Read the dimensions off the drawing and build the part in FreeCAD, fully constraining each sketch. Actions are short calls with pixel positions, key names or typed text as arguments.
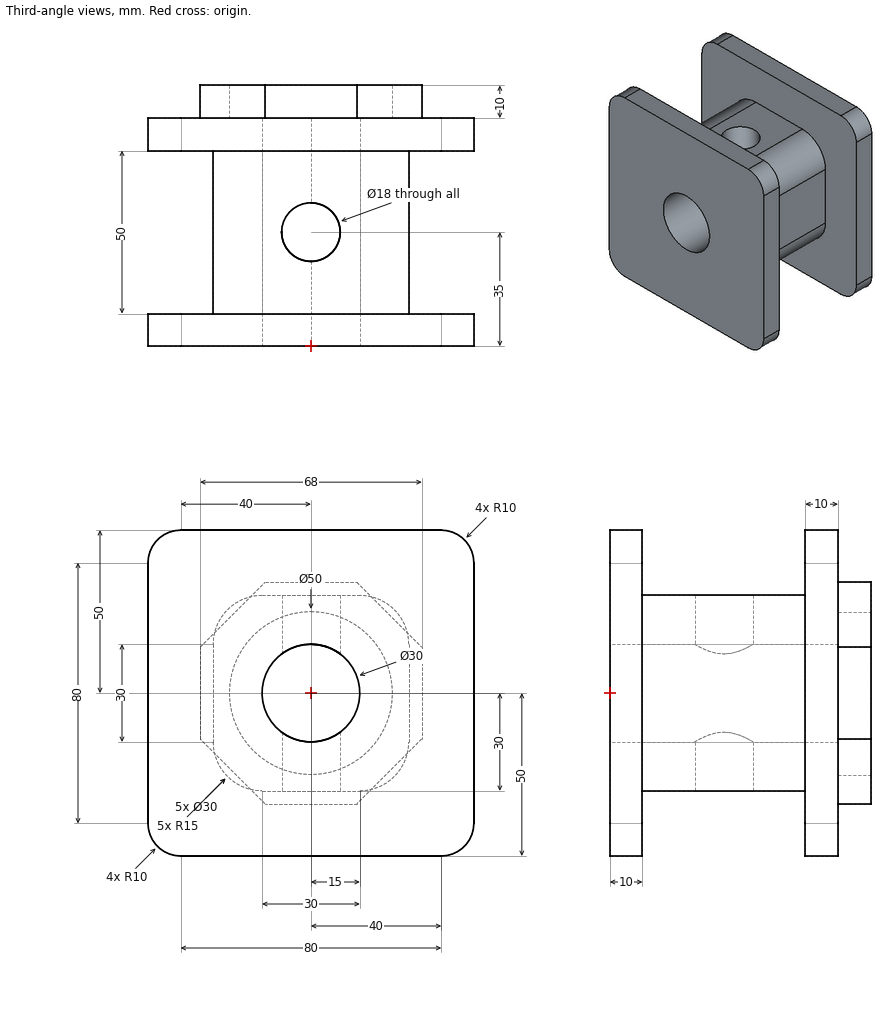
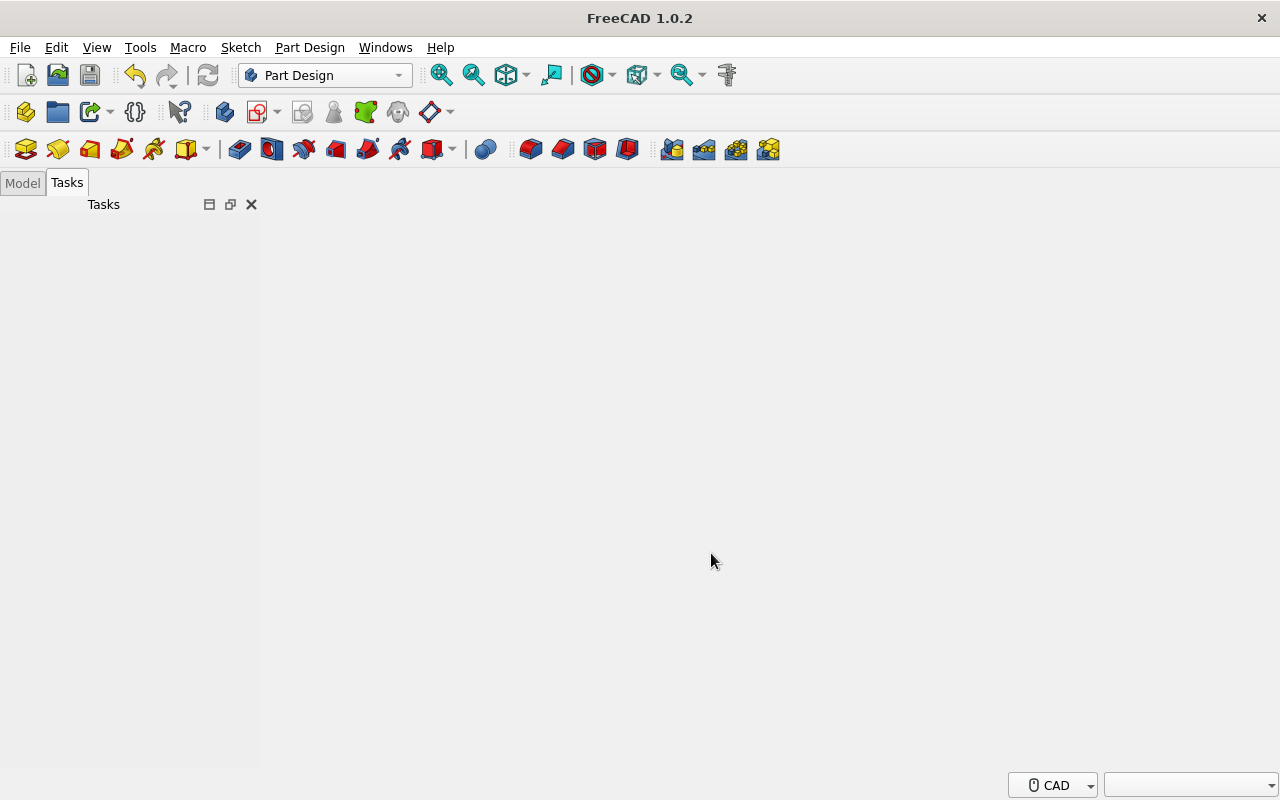
click(26, 76)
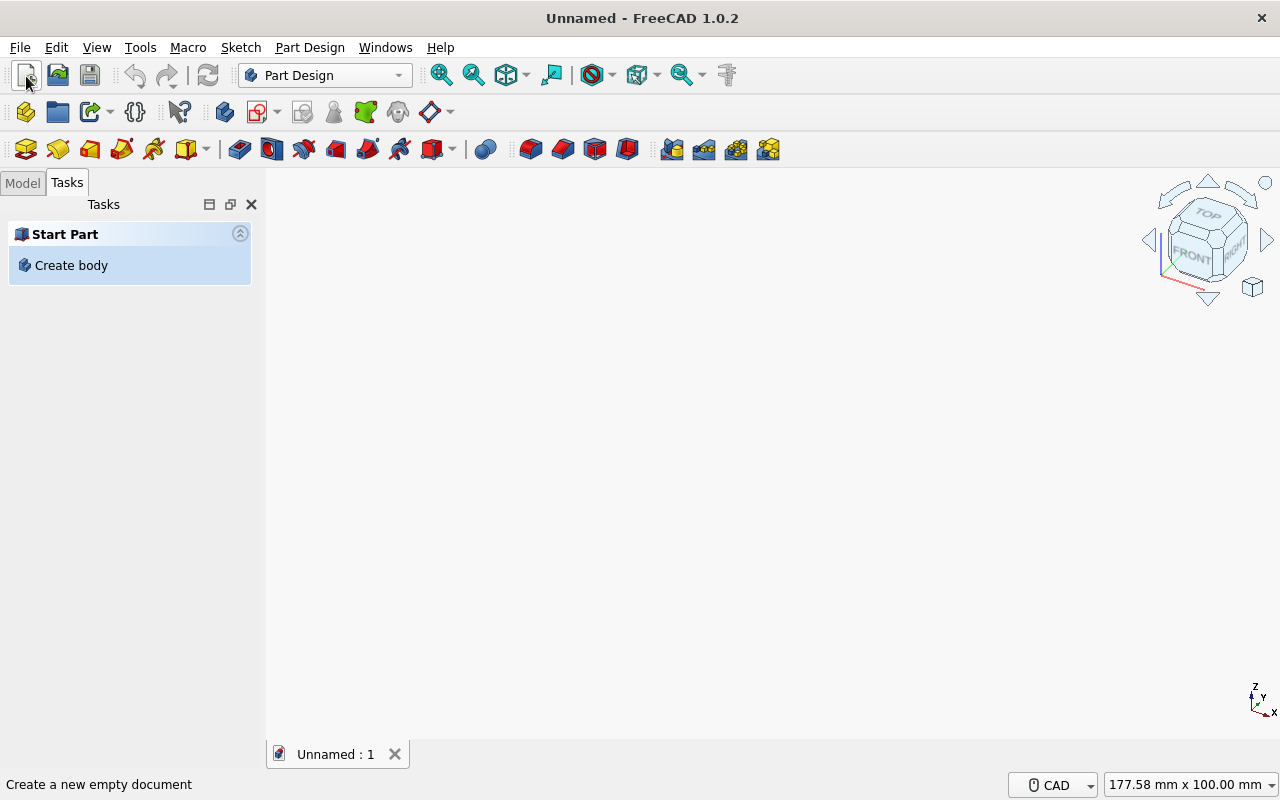
click(258, 112)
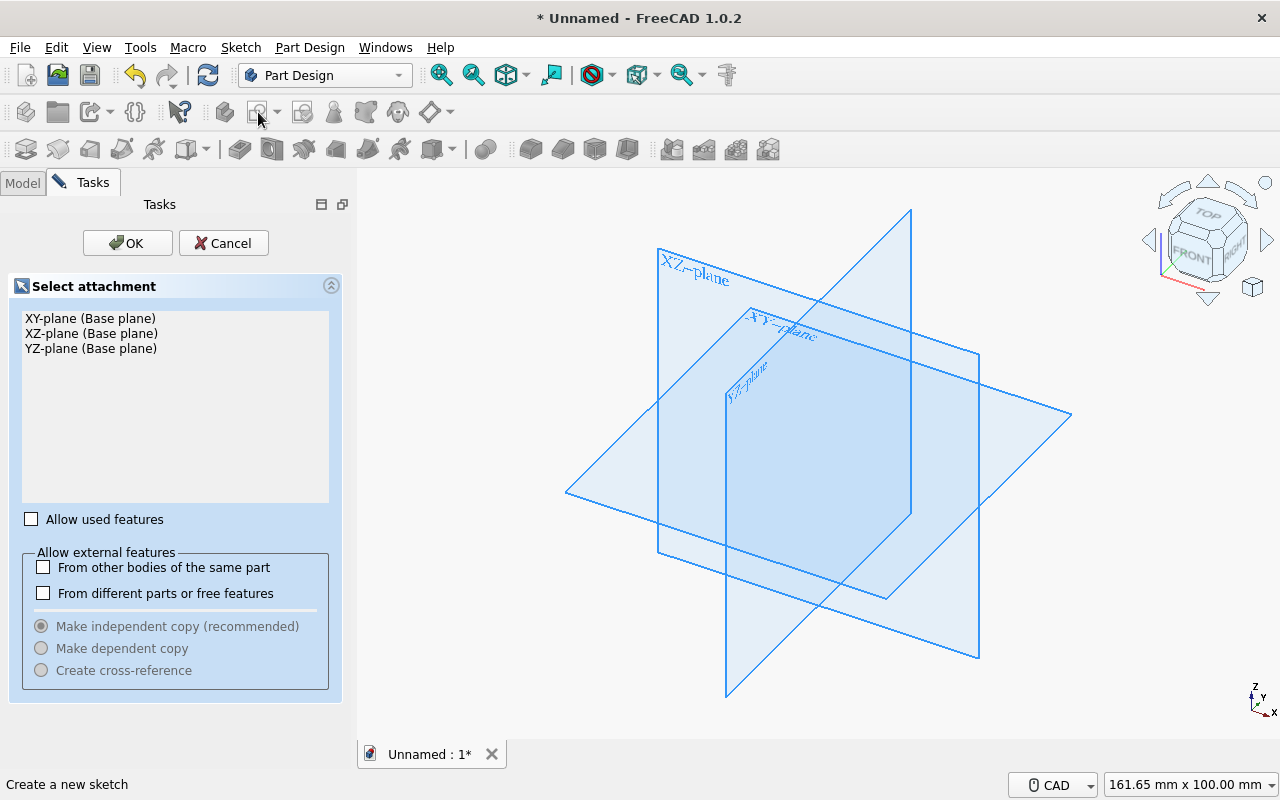
click(82, 334)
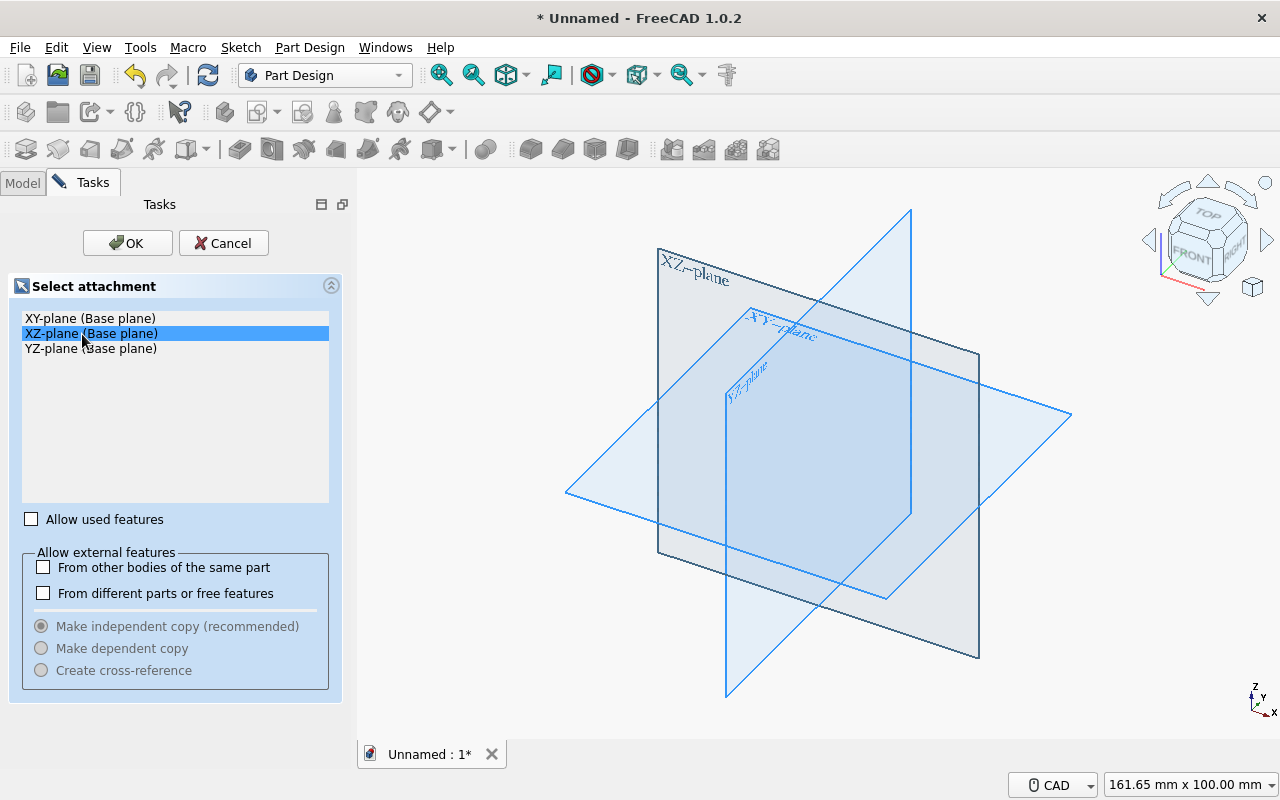
click(128, 243)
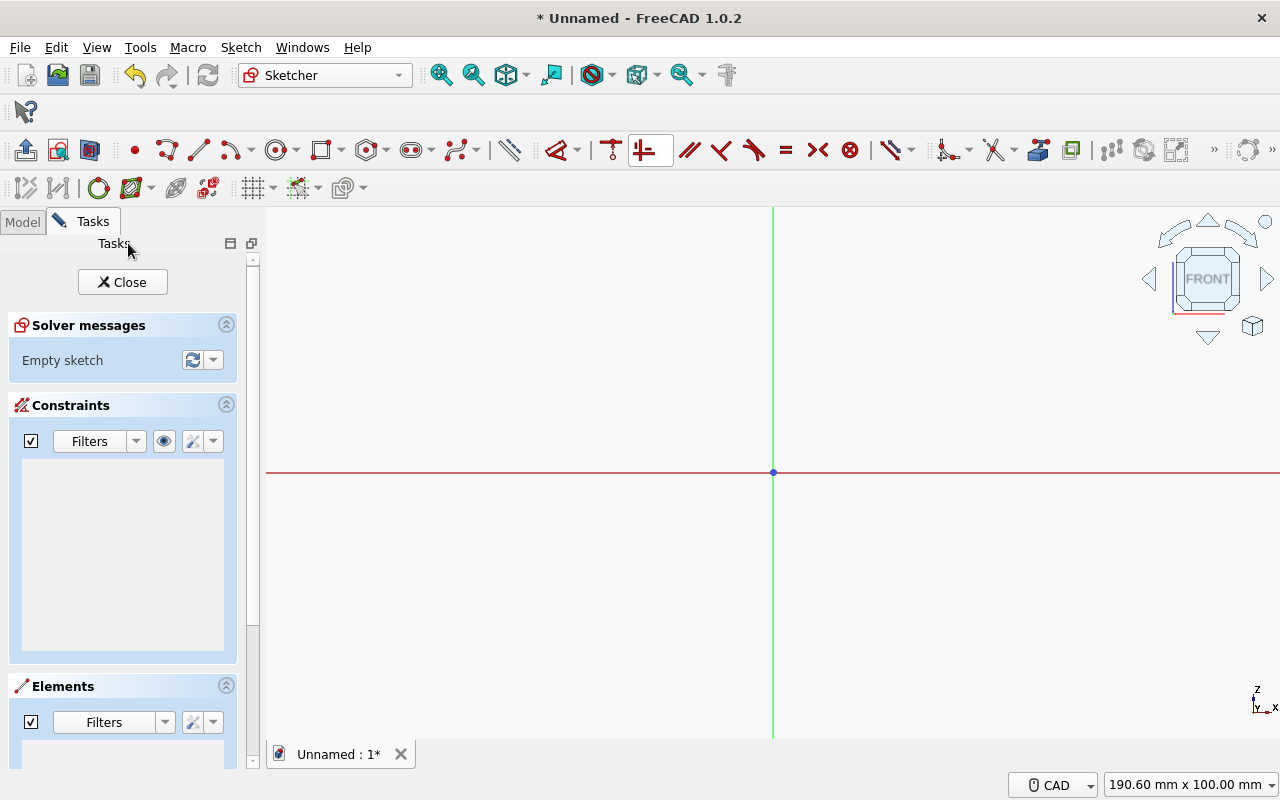
scroll(565, 473, down, 2)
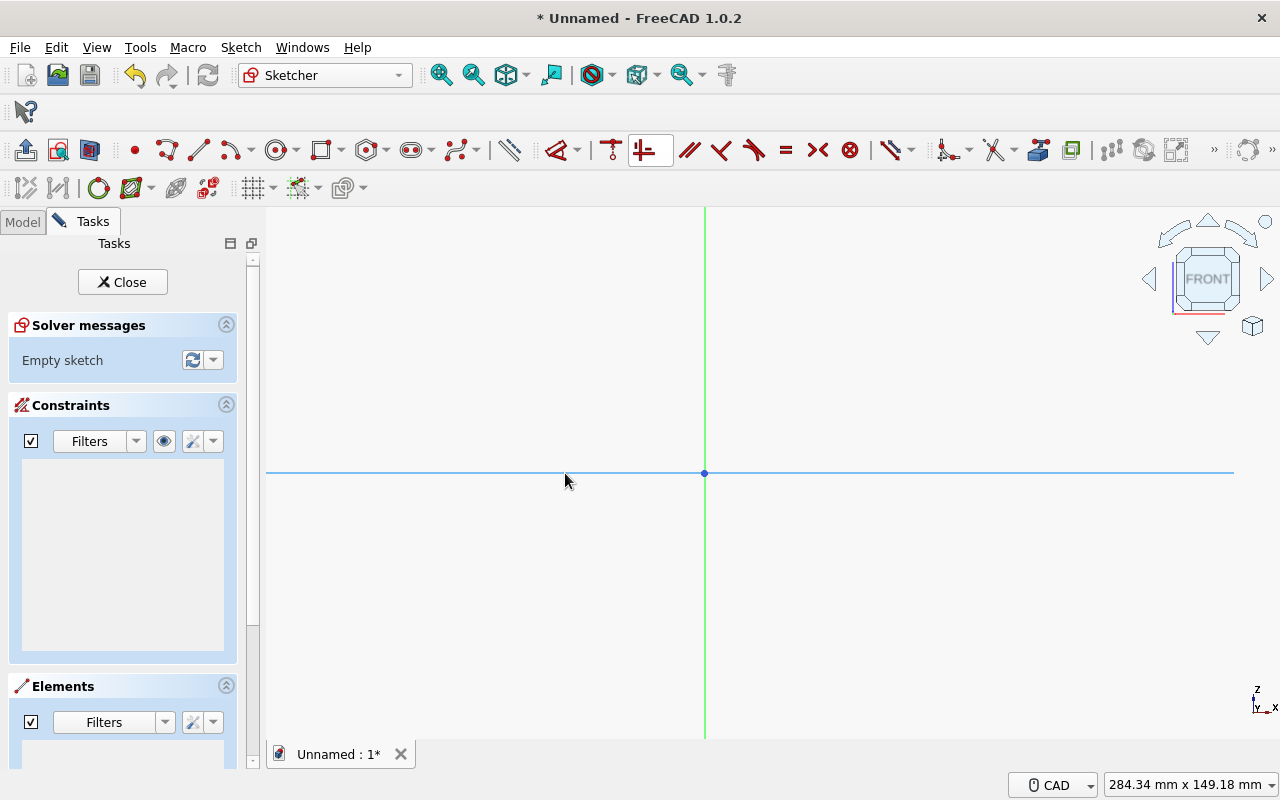
click(200, 150)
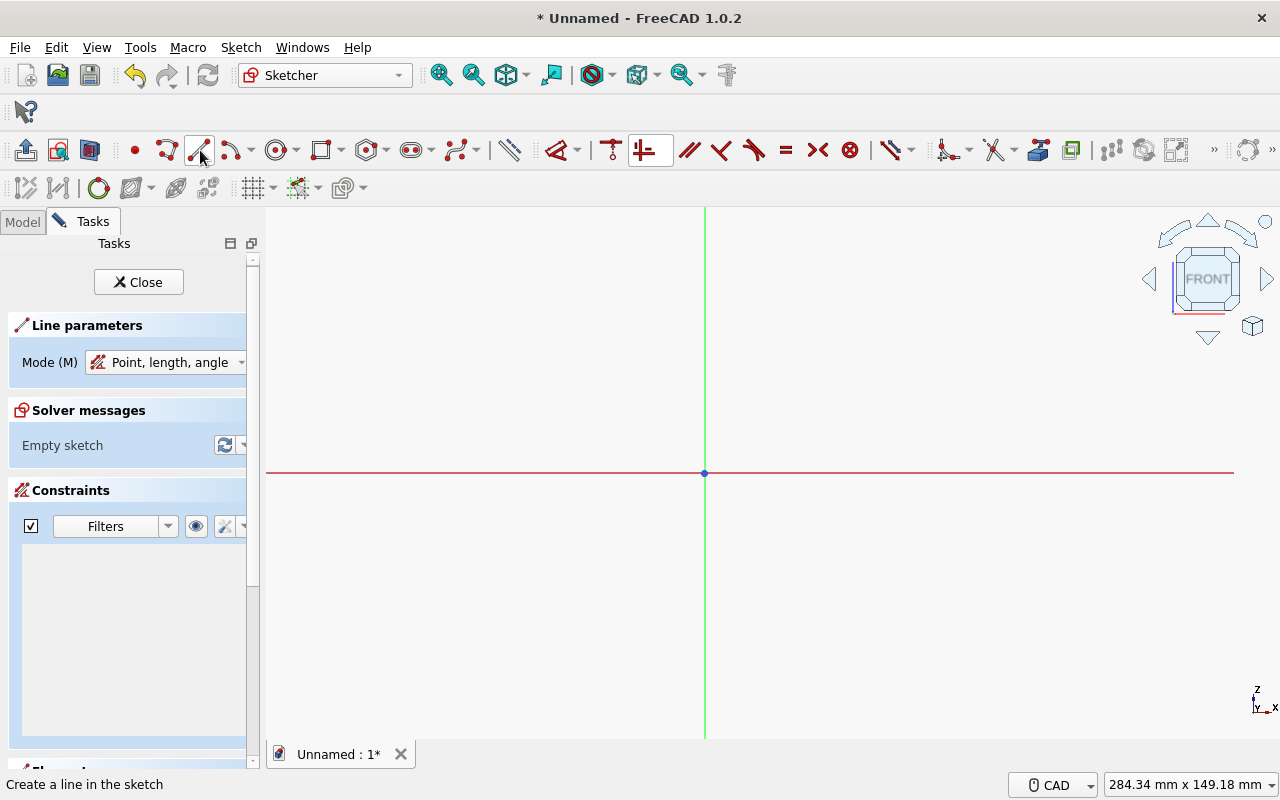
click(847, 651)
click(562, 651)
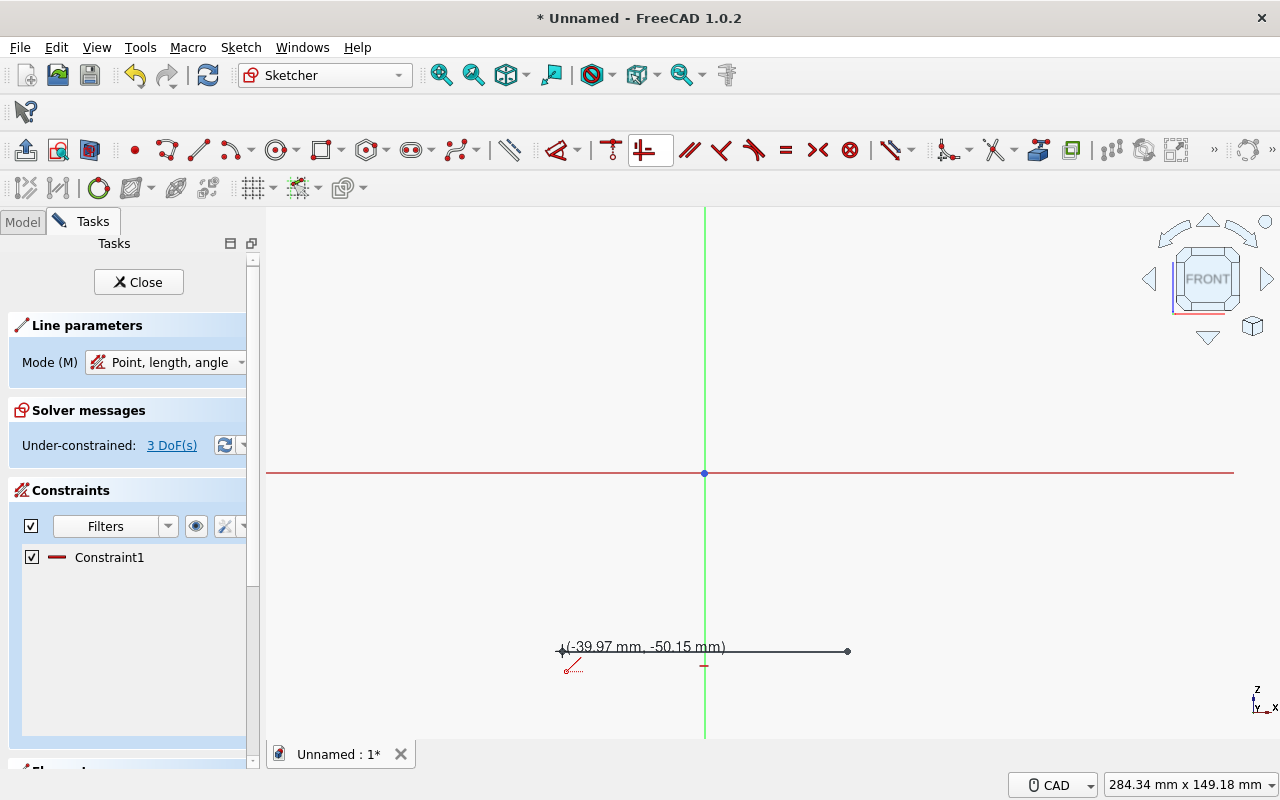
click(526, 616)
click(526, 331)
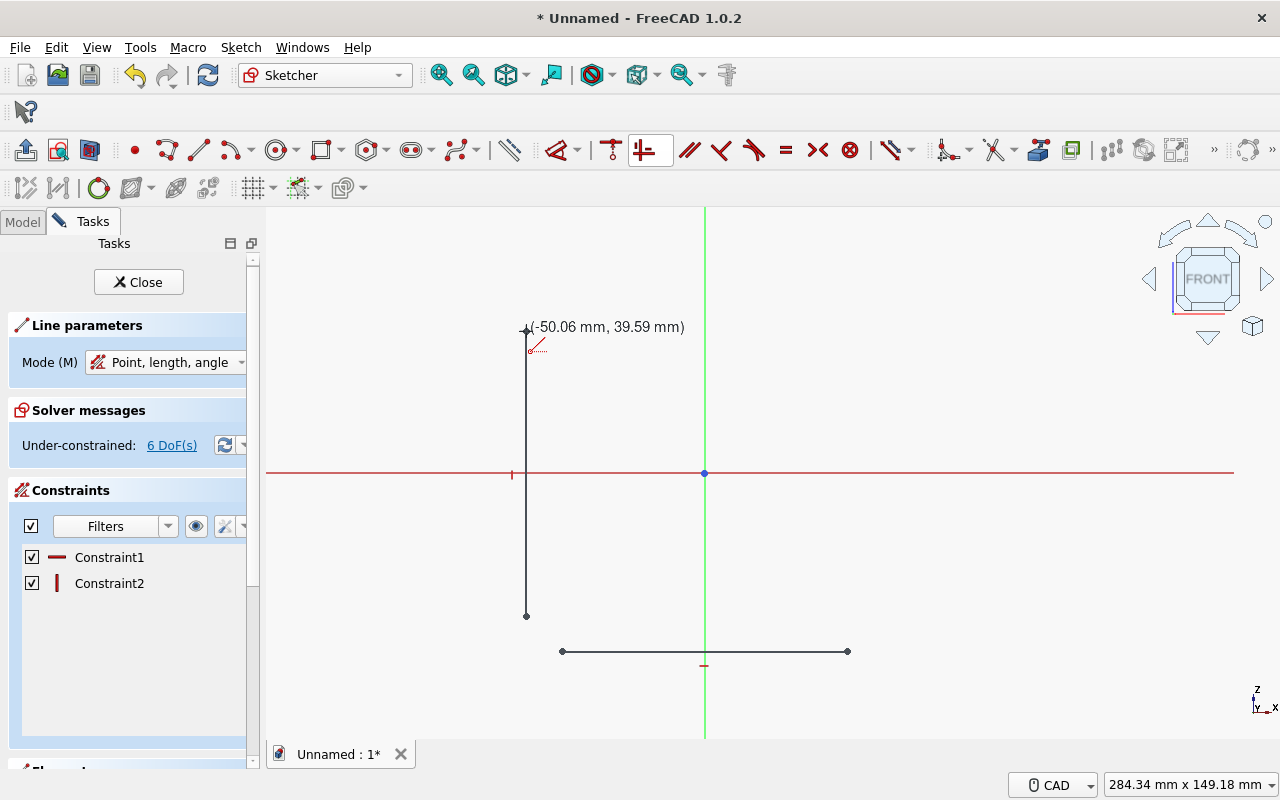
click(562, 295)
click(847, 295)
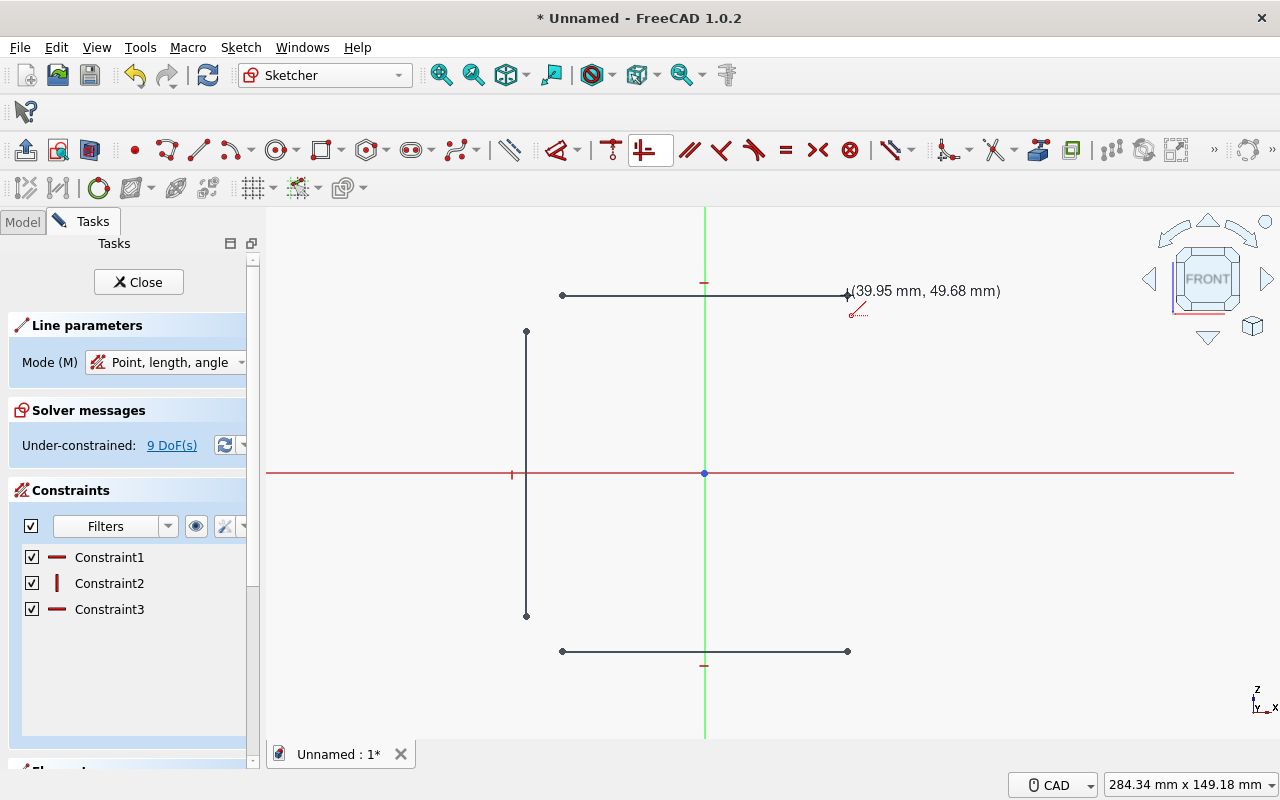
click(883, 331)
click(883, 616)